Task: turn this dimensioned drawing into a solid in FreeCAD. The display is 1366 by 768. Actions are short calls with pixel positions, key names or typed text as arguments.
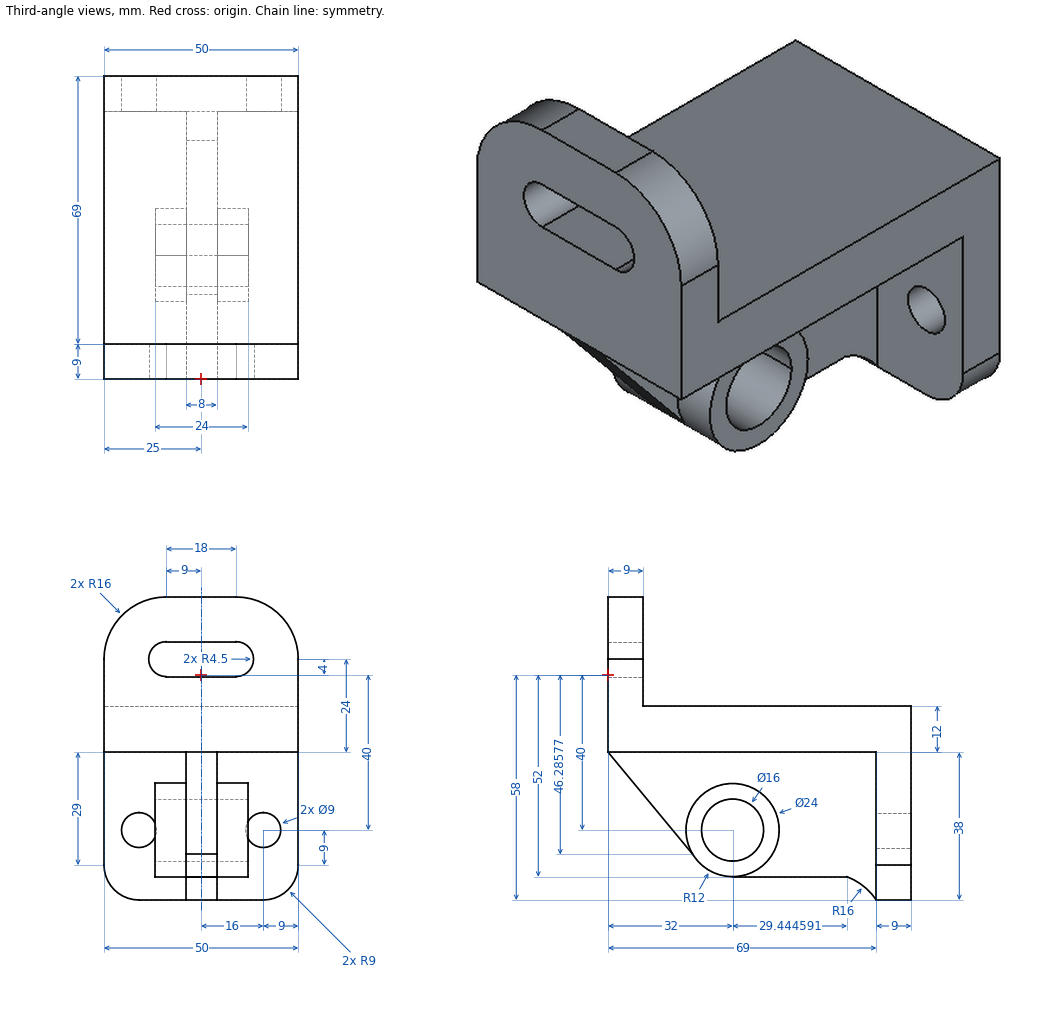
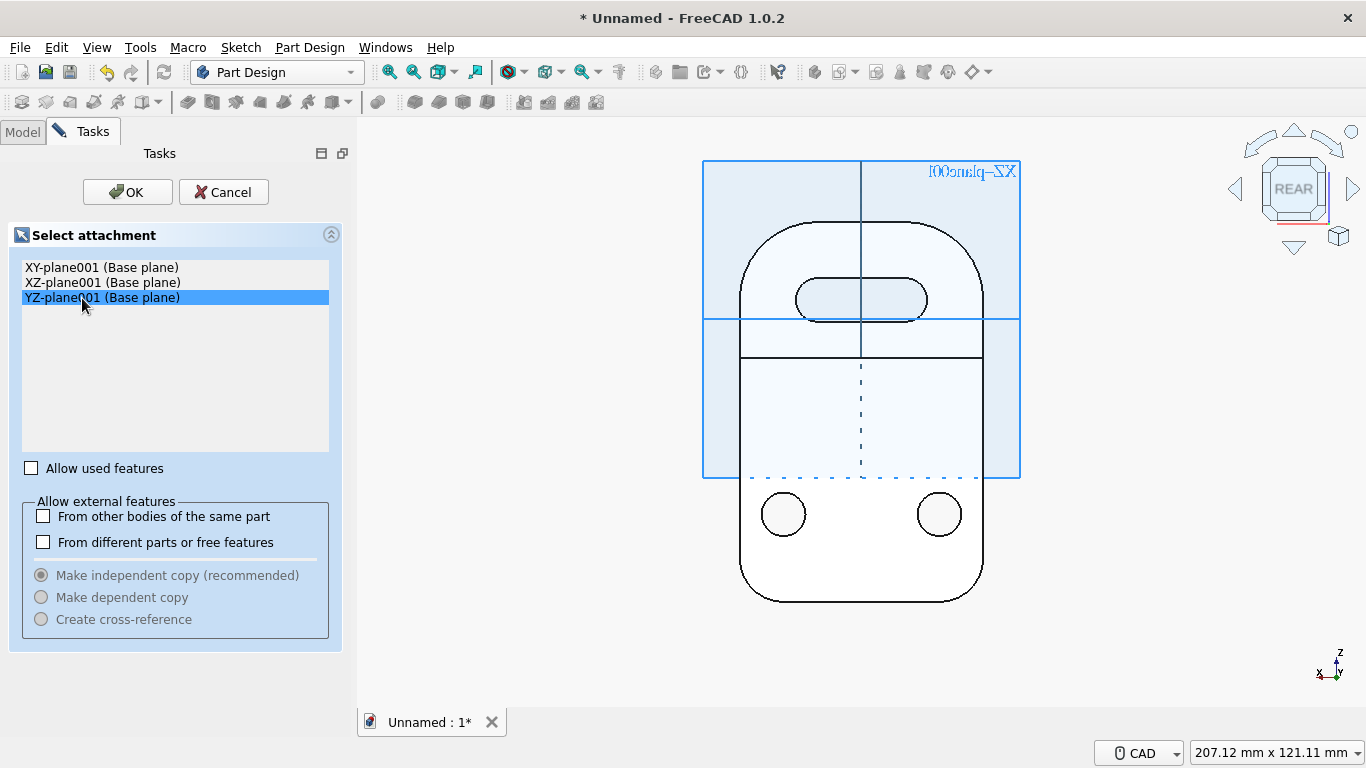
click(128, 192)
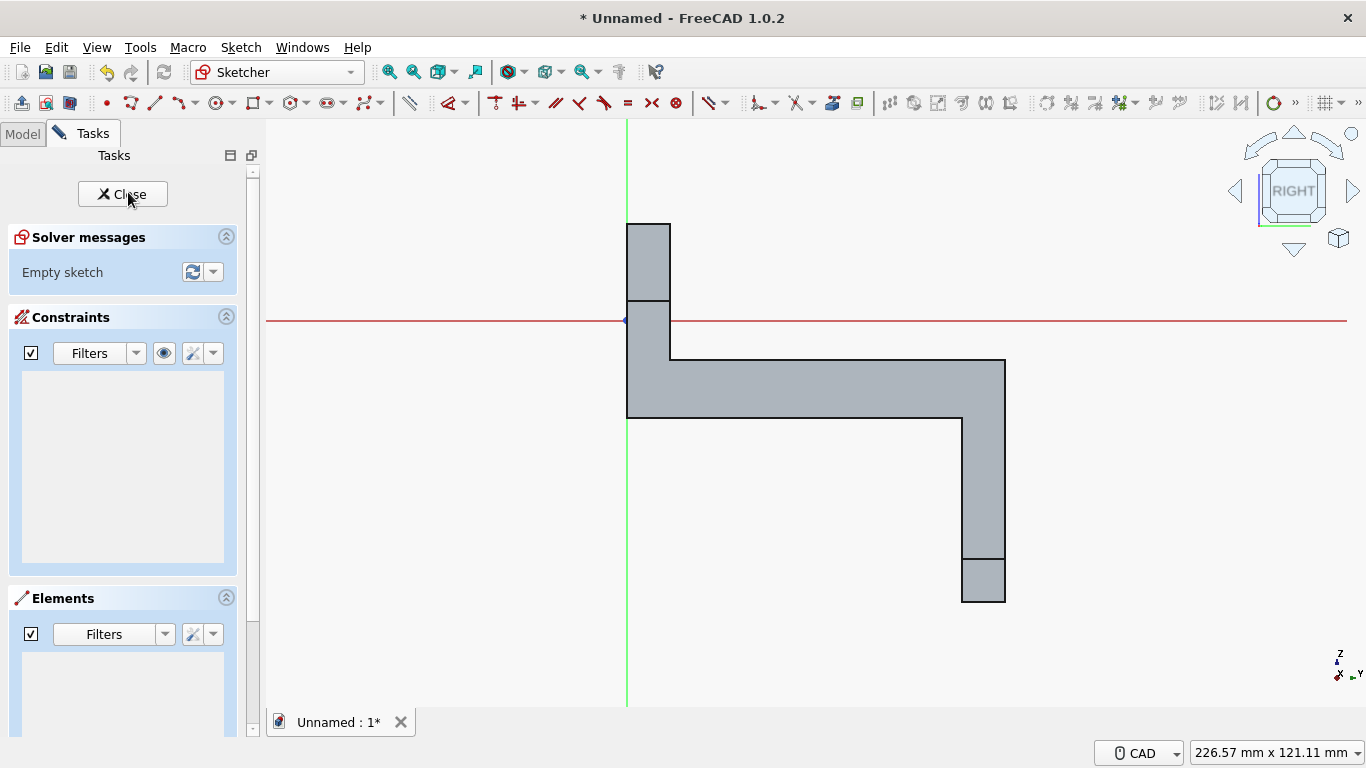
scroll(705, 516, up, 2)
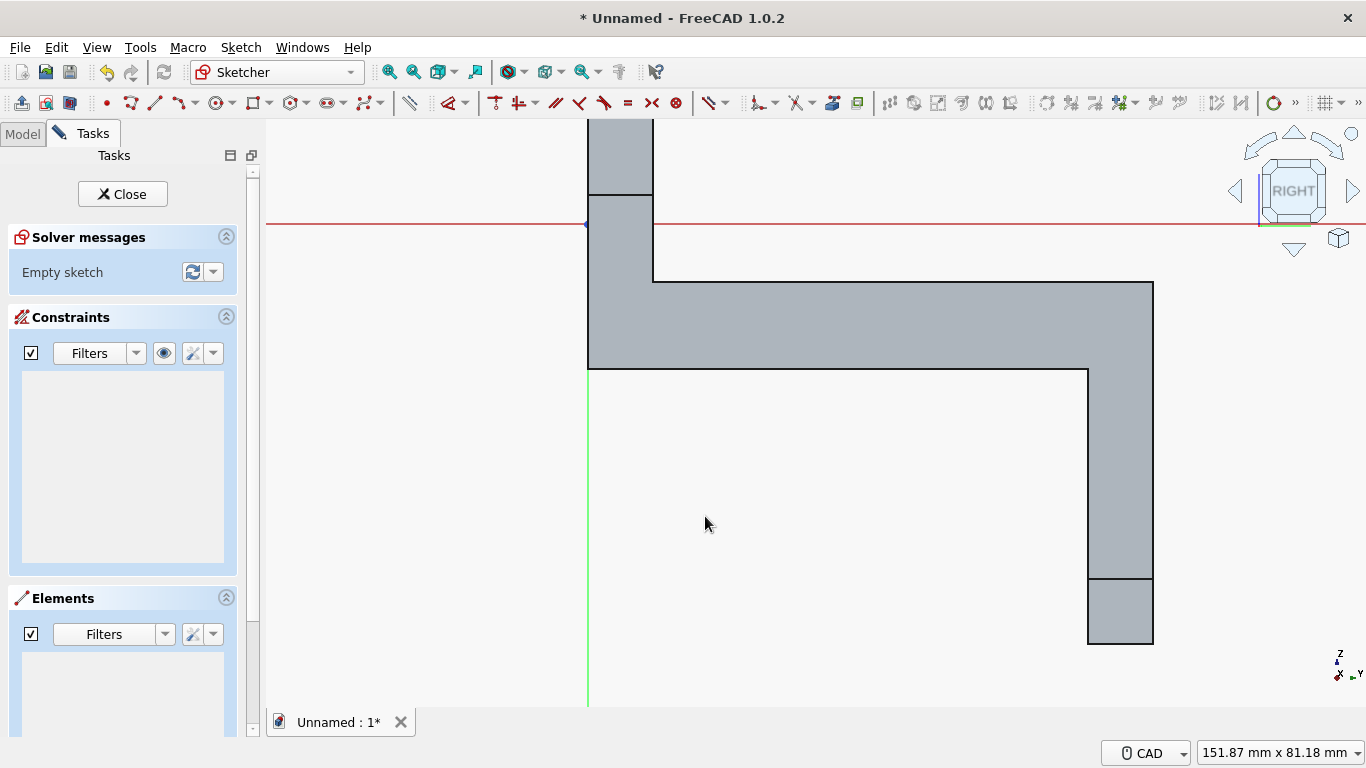
click(216, 104)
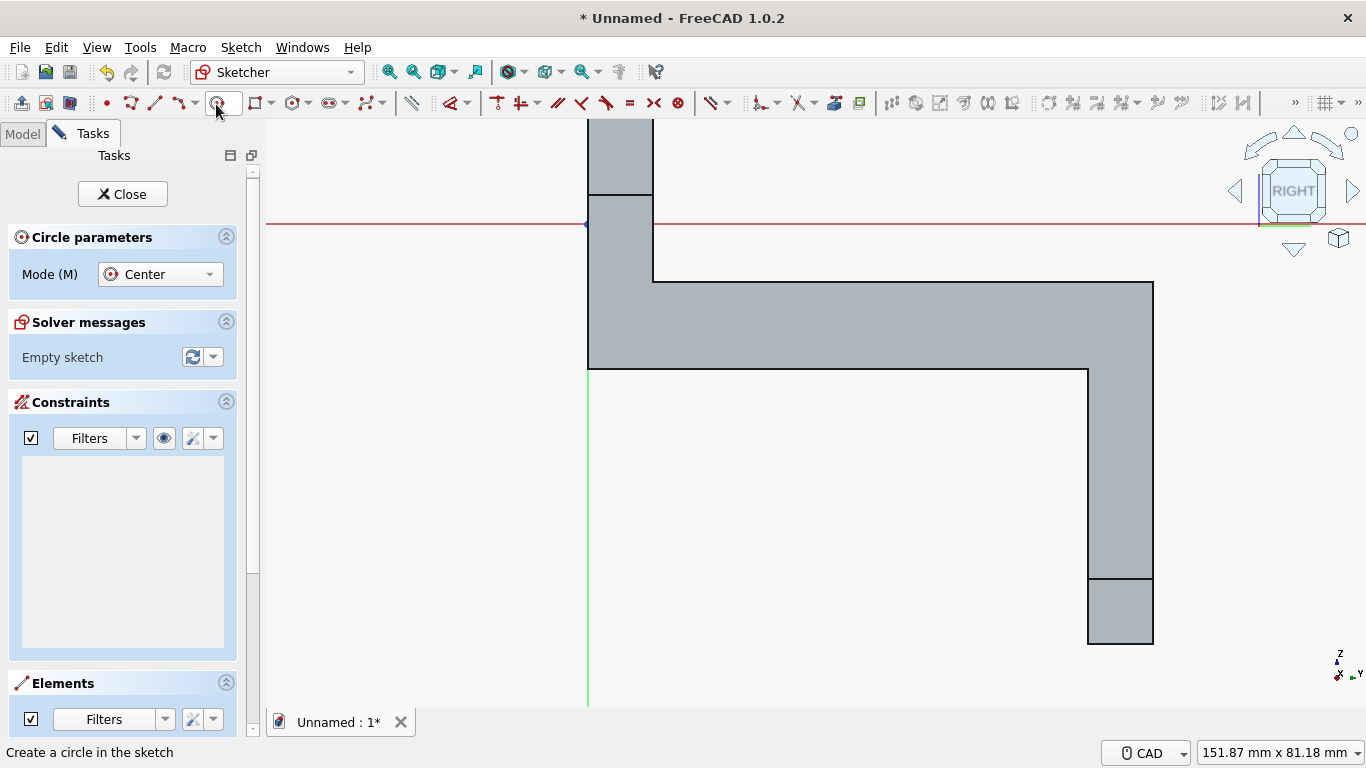
click(820, 514)
click(881, 453)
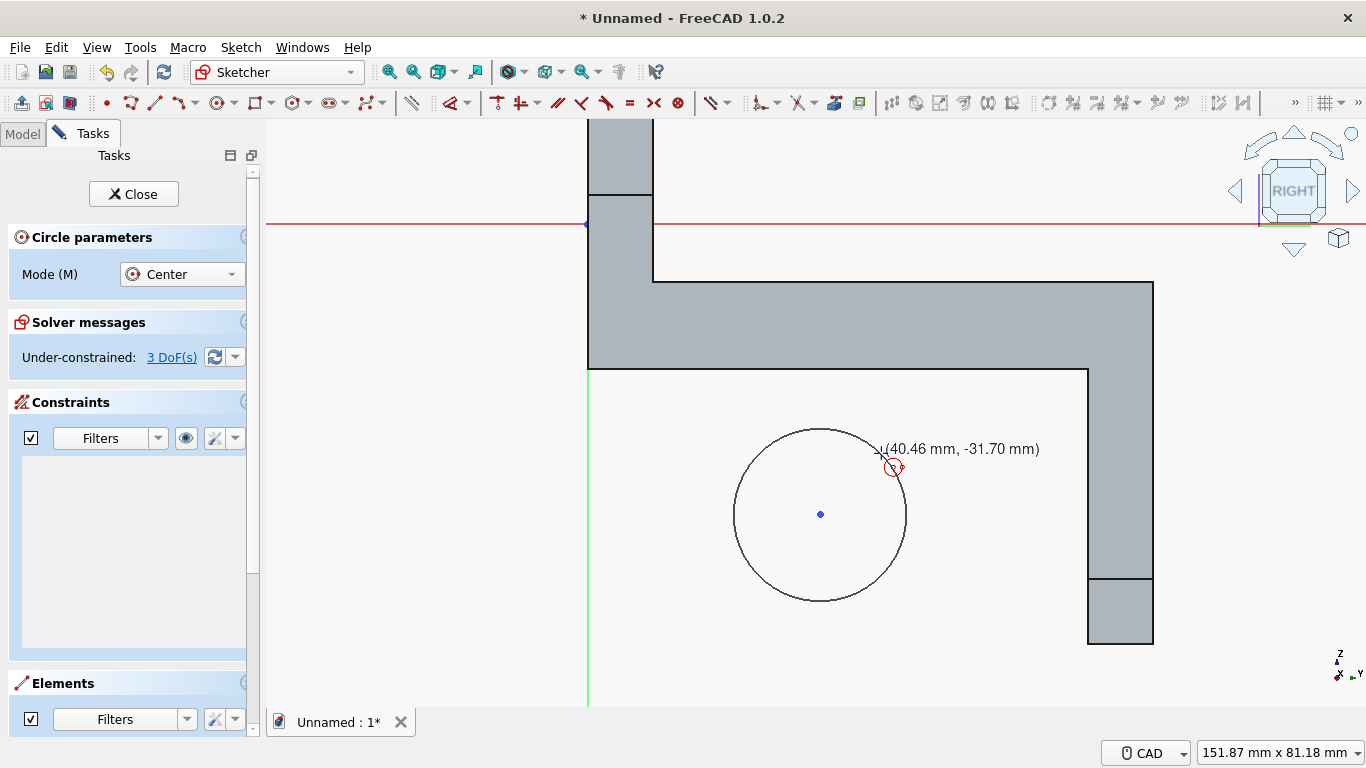
click(820, 515)
click(861, 473)
key(Escape)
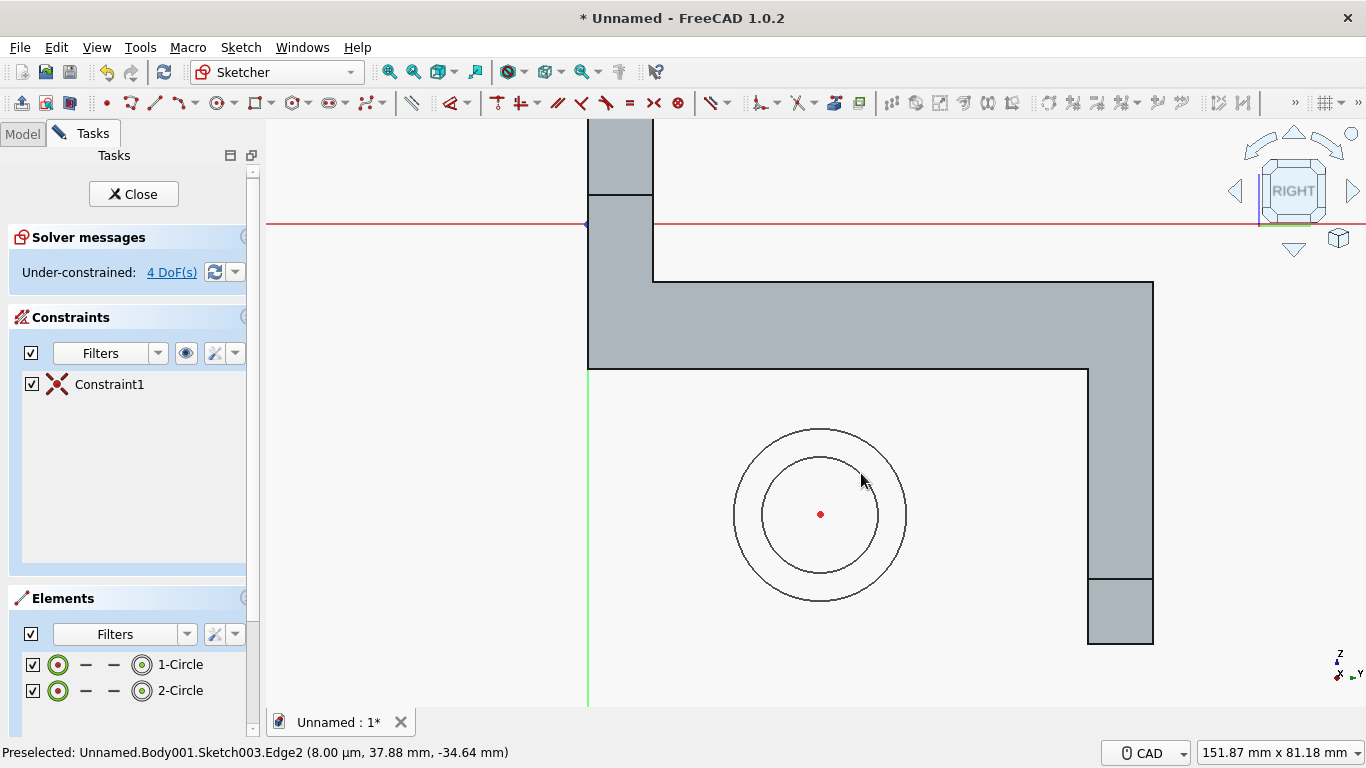
click(450, 104)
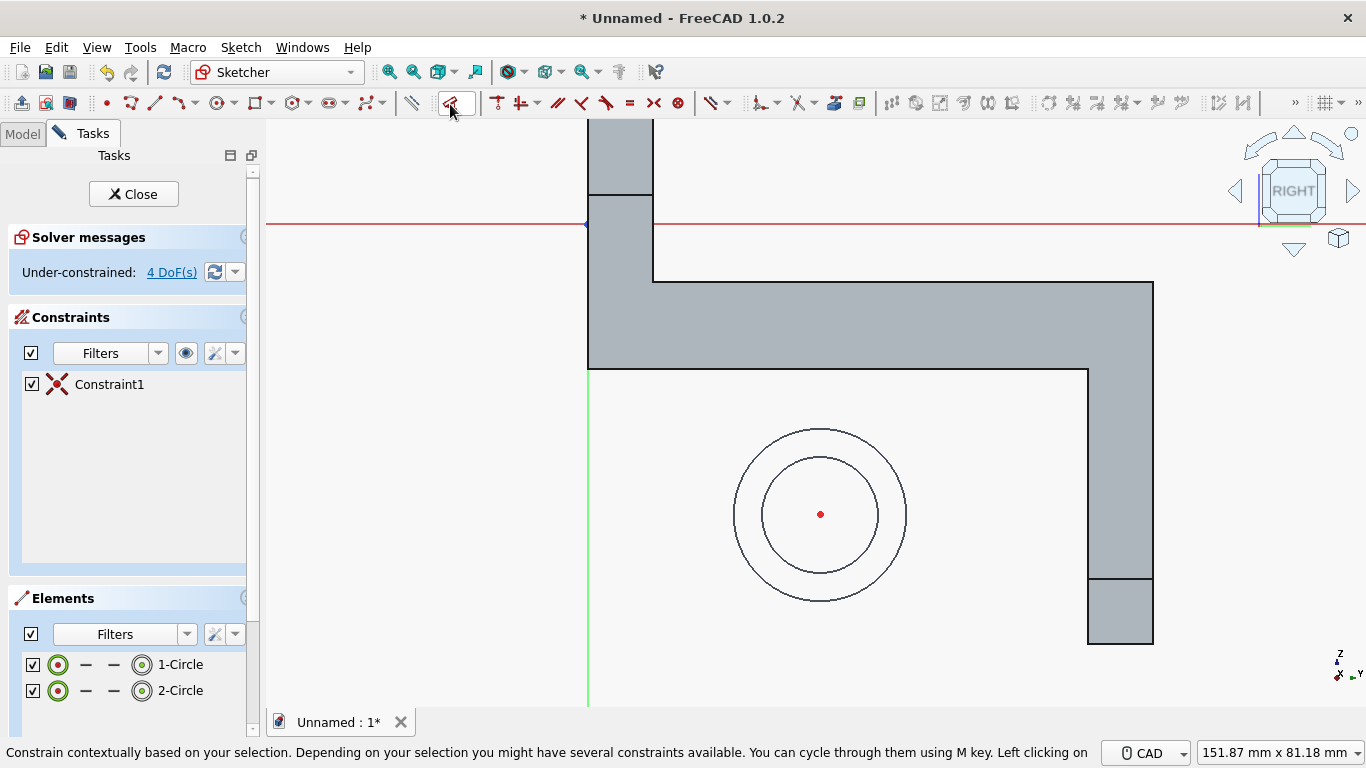
click(881, 454)
click(904, 431)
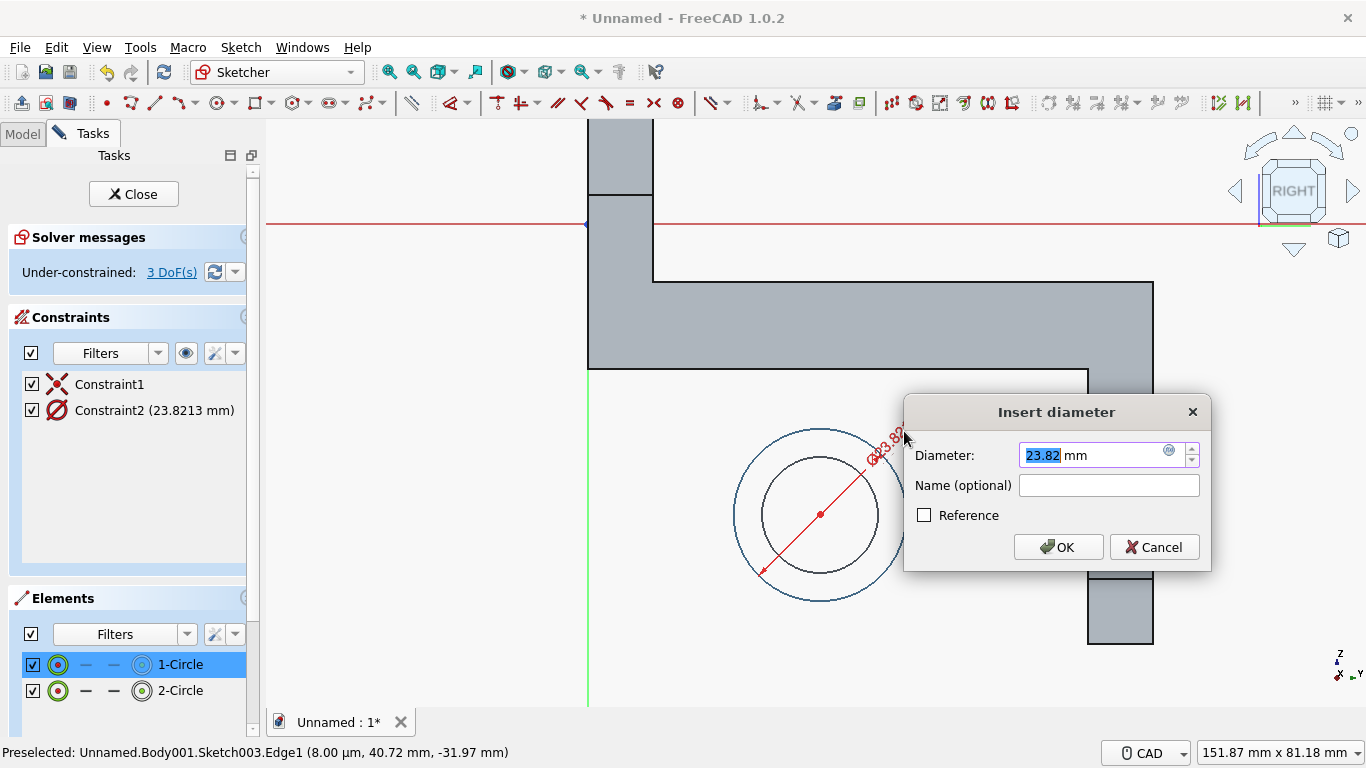
text(24)
key(Return)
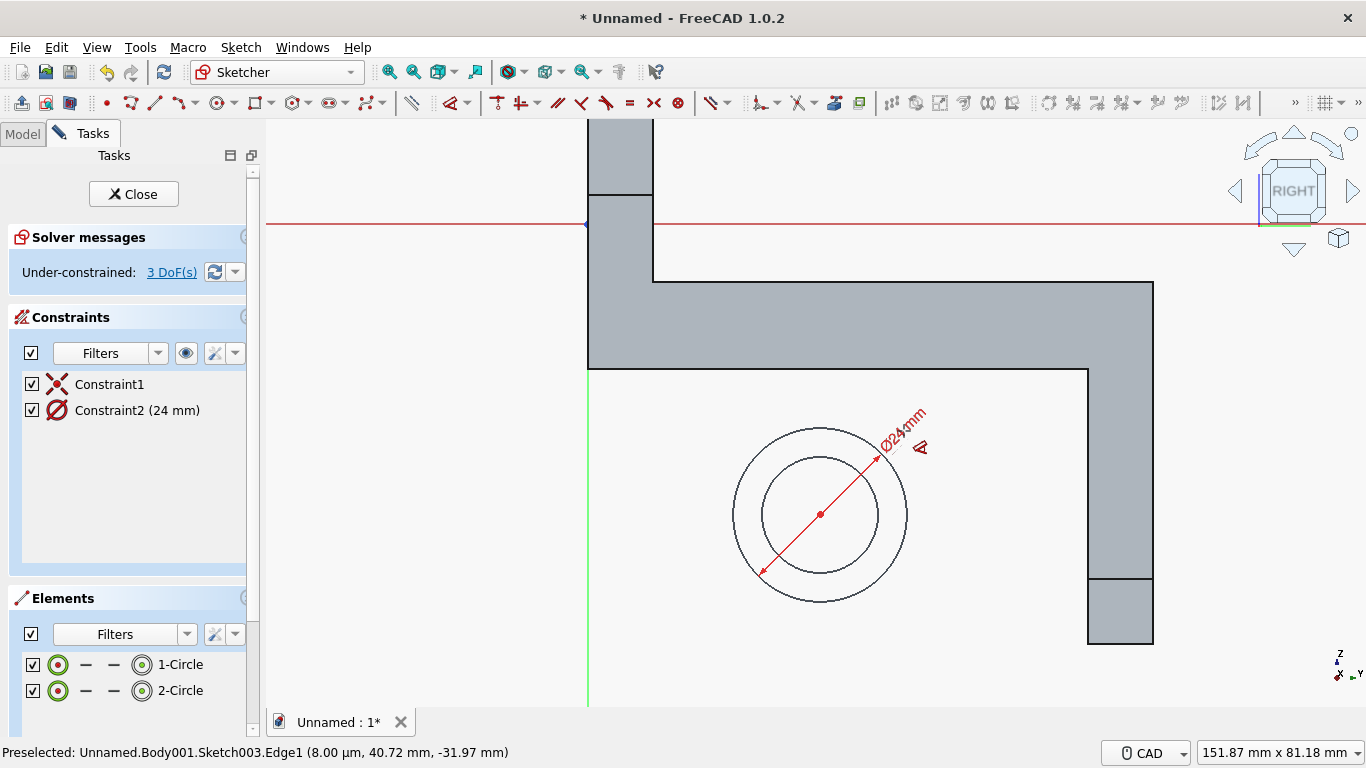
click(861, 474)
click(928, 483)